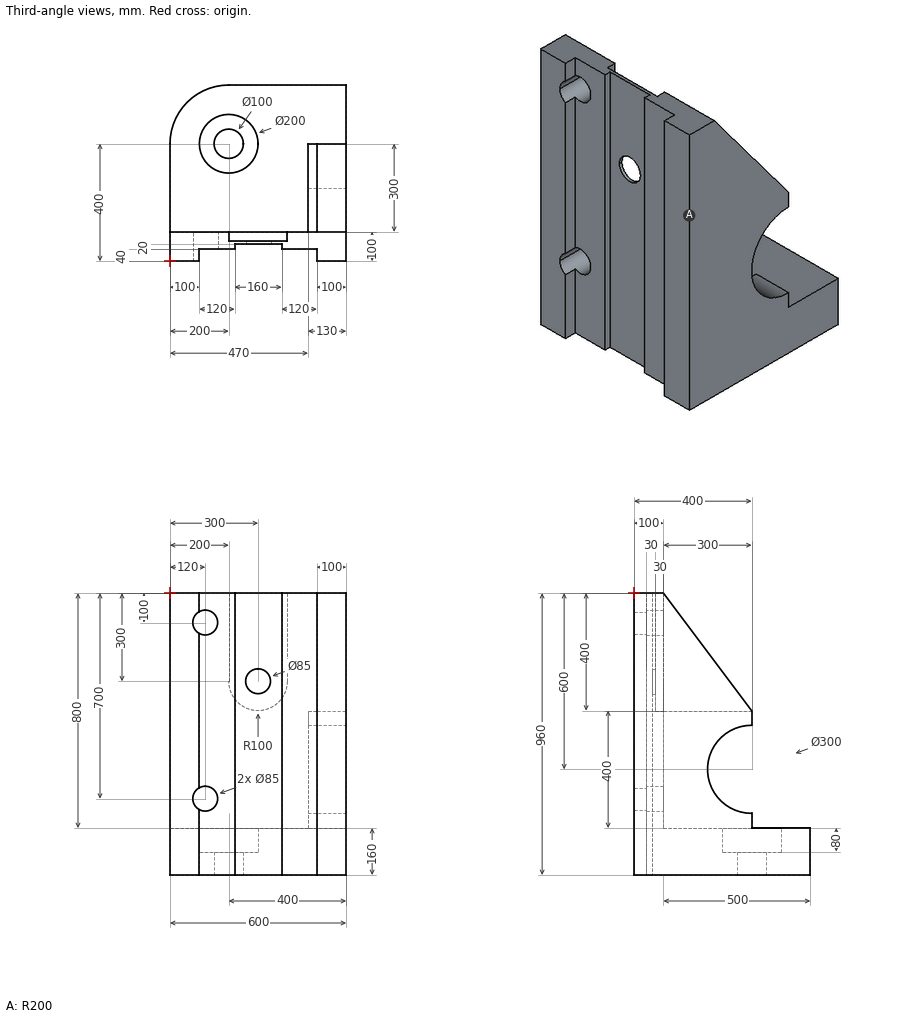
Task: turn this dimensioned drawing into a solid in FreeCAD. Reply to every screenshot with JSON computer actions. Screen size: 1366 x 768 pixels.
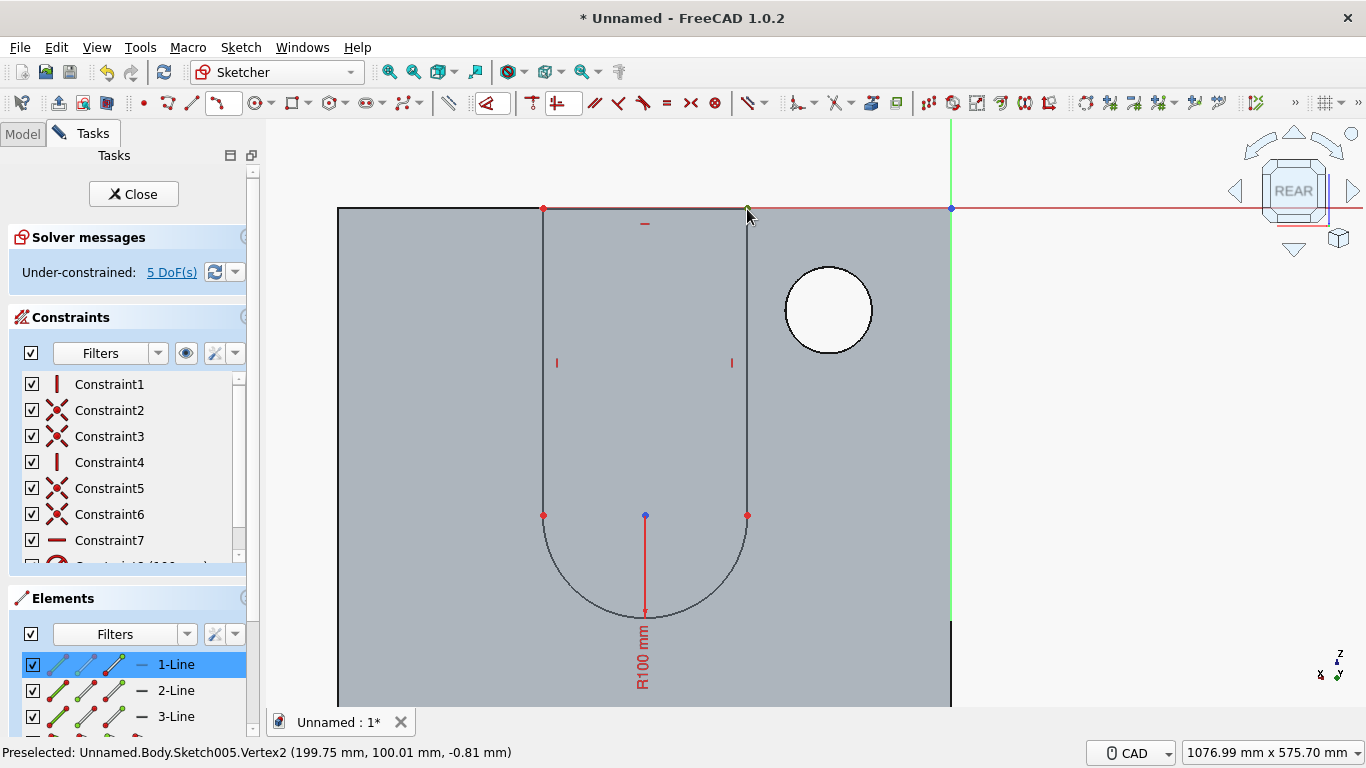
{"action": "left_click", "coordinate": [812, 208]}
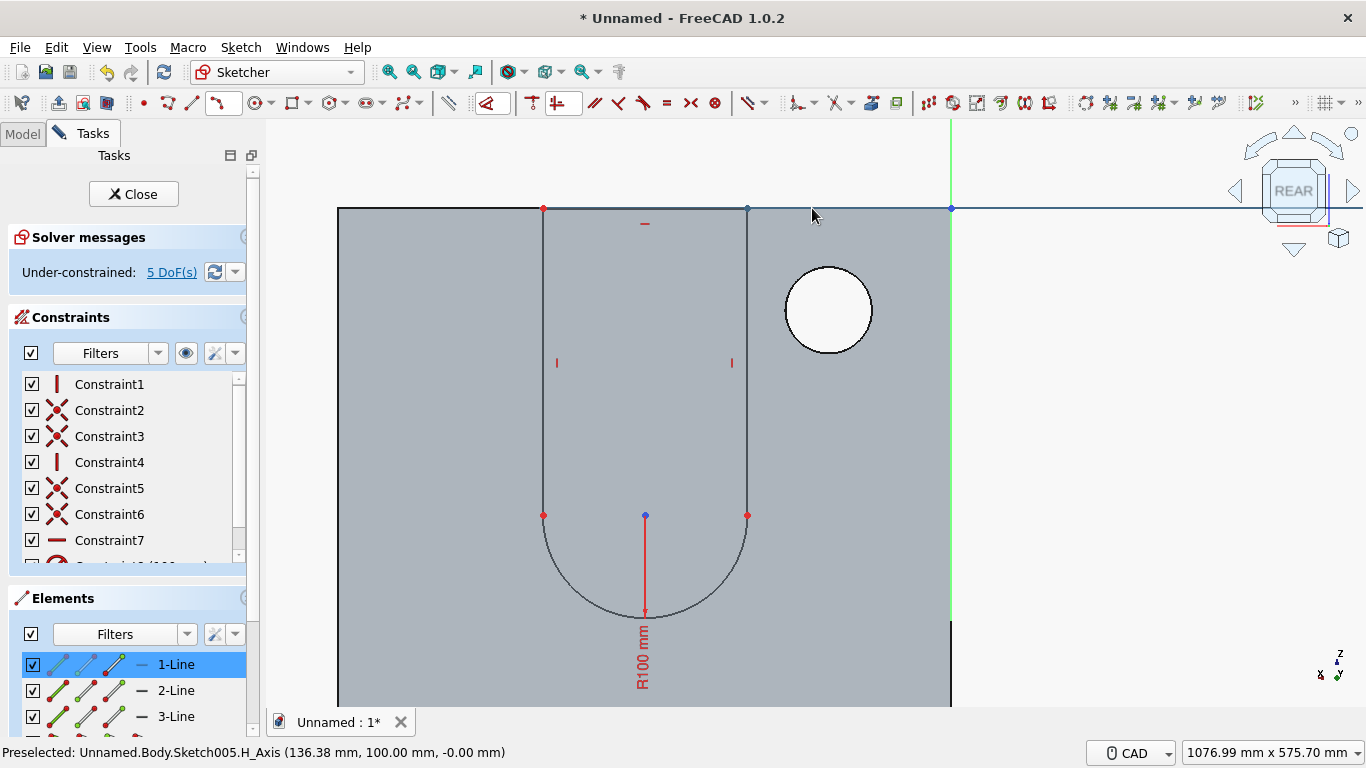
{"action": "left_click", "coordinate": [532, 104]}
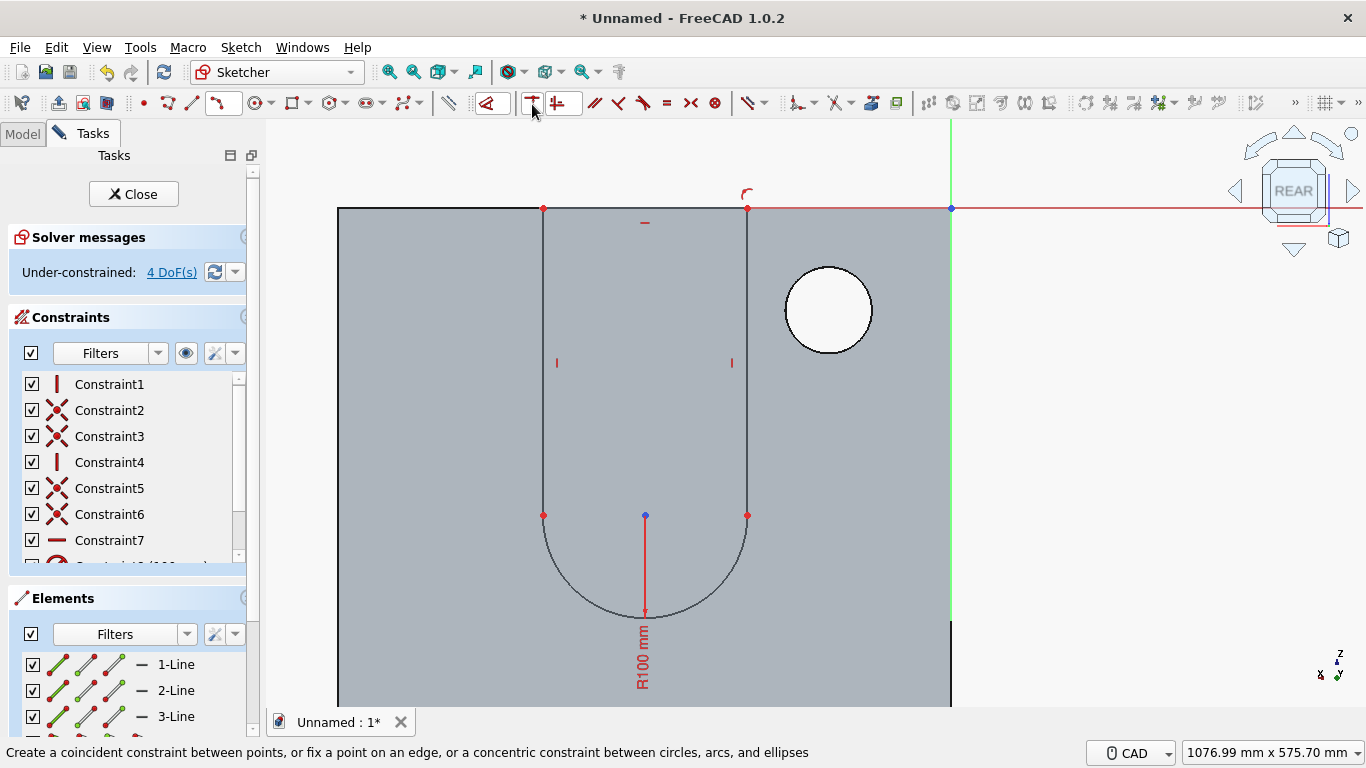
{"action": "left_click", "coordinate": [747, 424]}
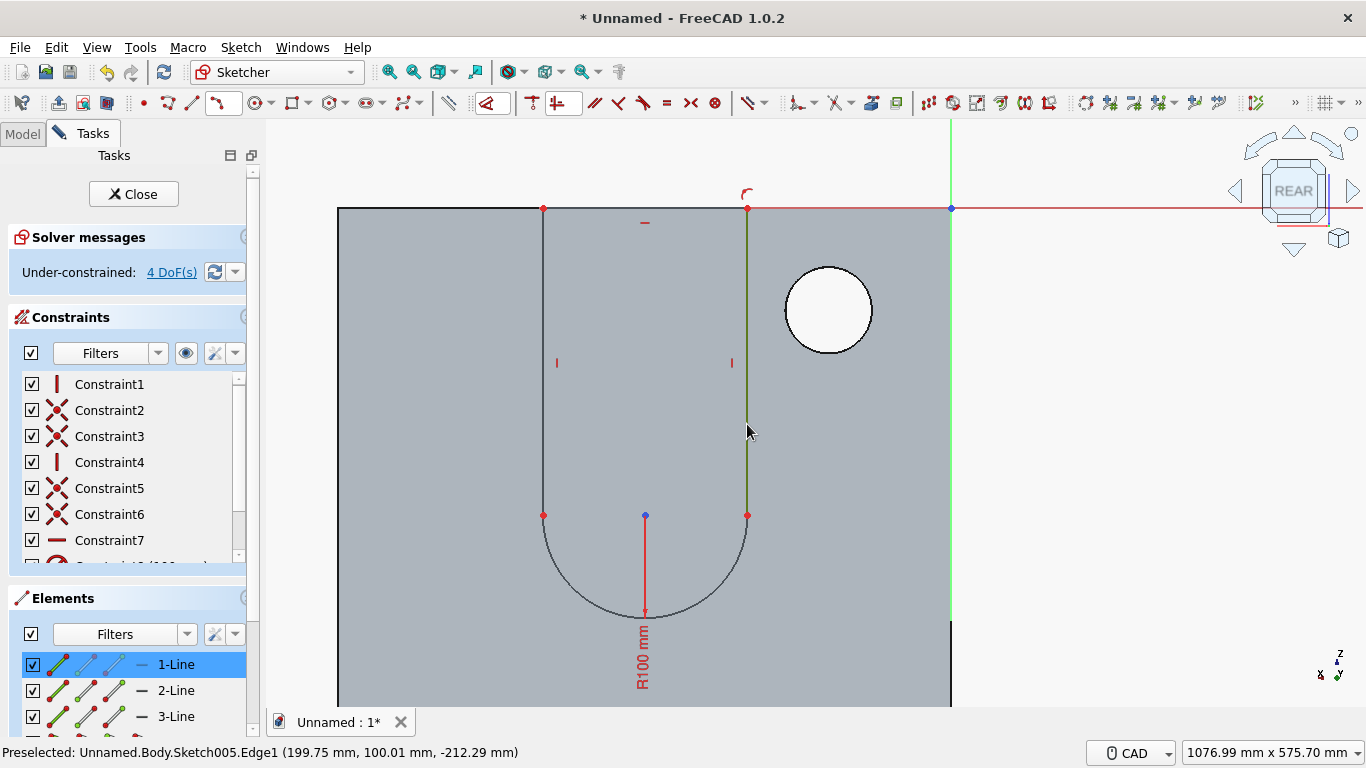
{"action": "key", "text": "i"}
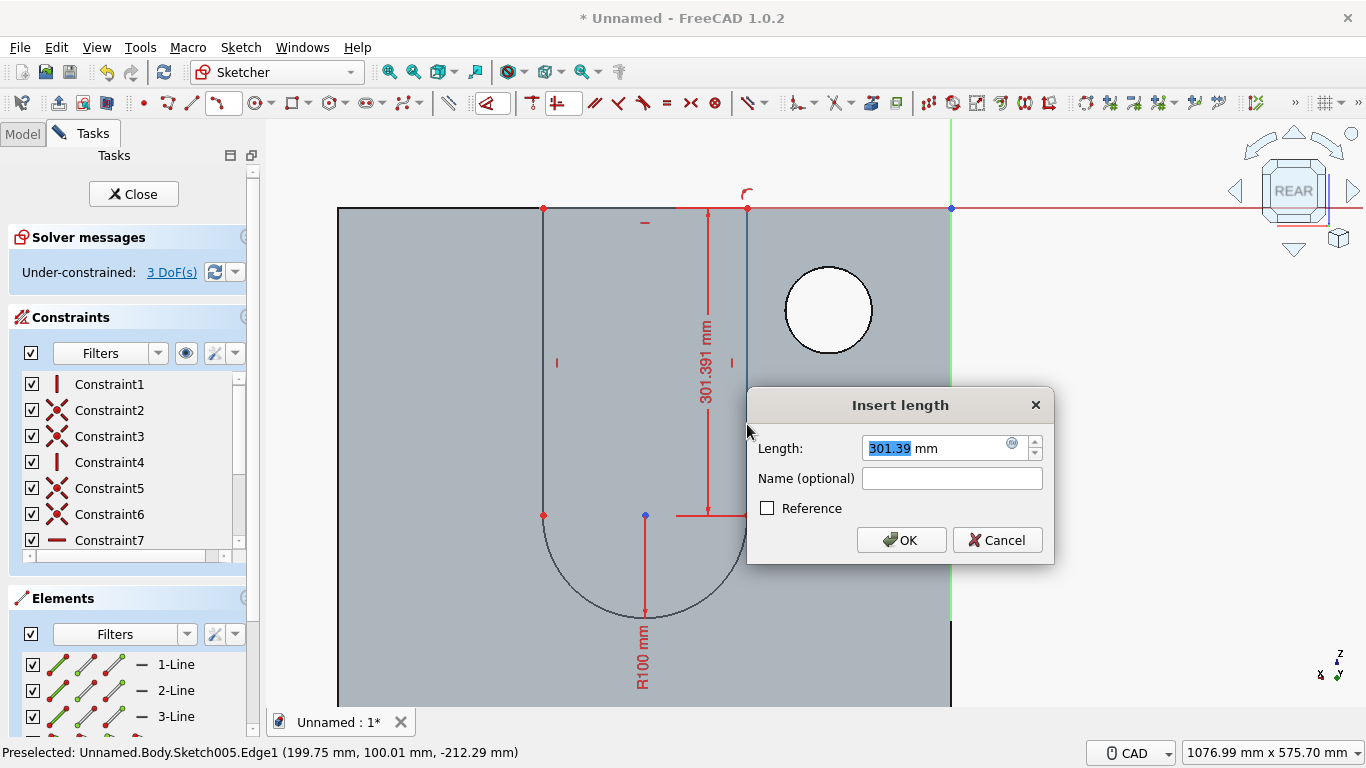
{"action": "type", "text": "300"}
{"action": "key", "text": "Return"}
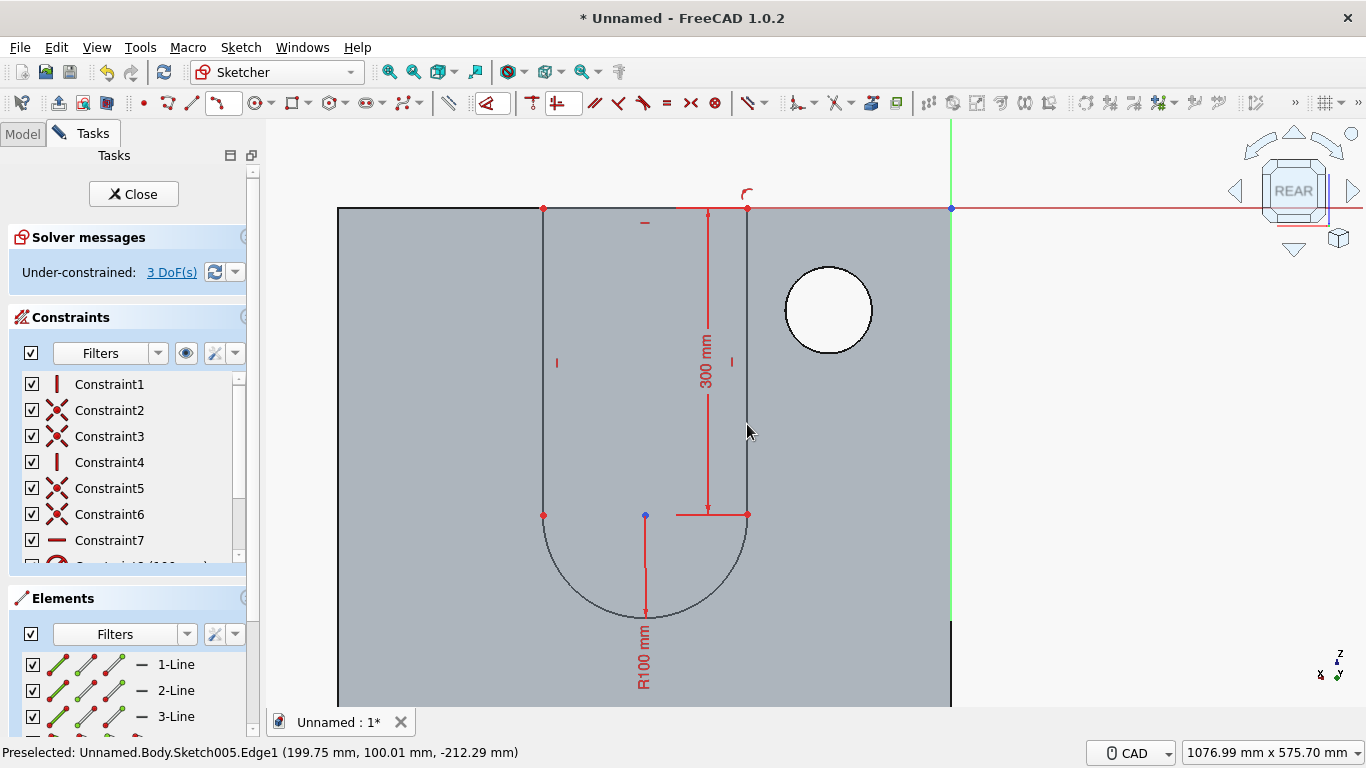
{"action": "left_click", "coordinate": [543, 301]}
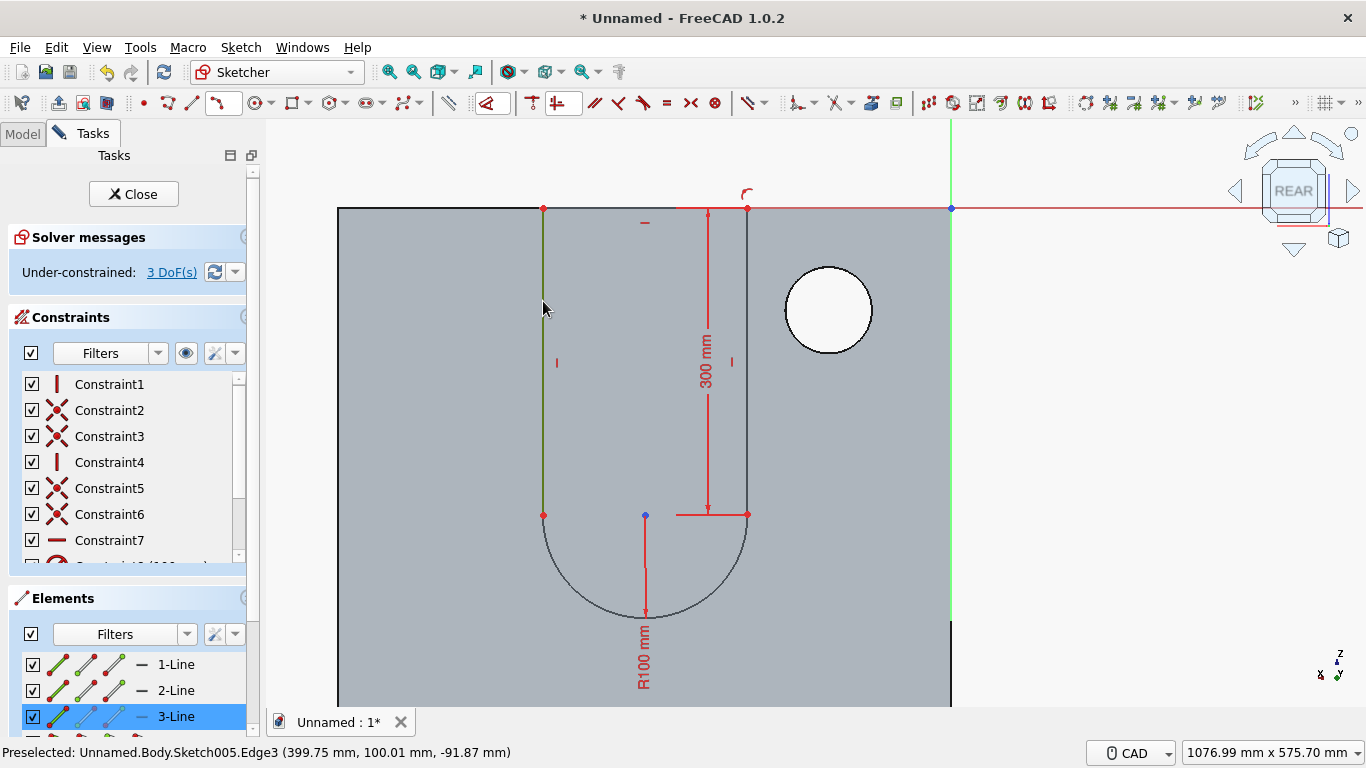
{"action": "left_click", "coordinate": [504, 104]}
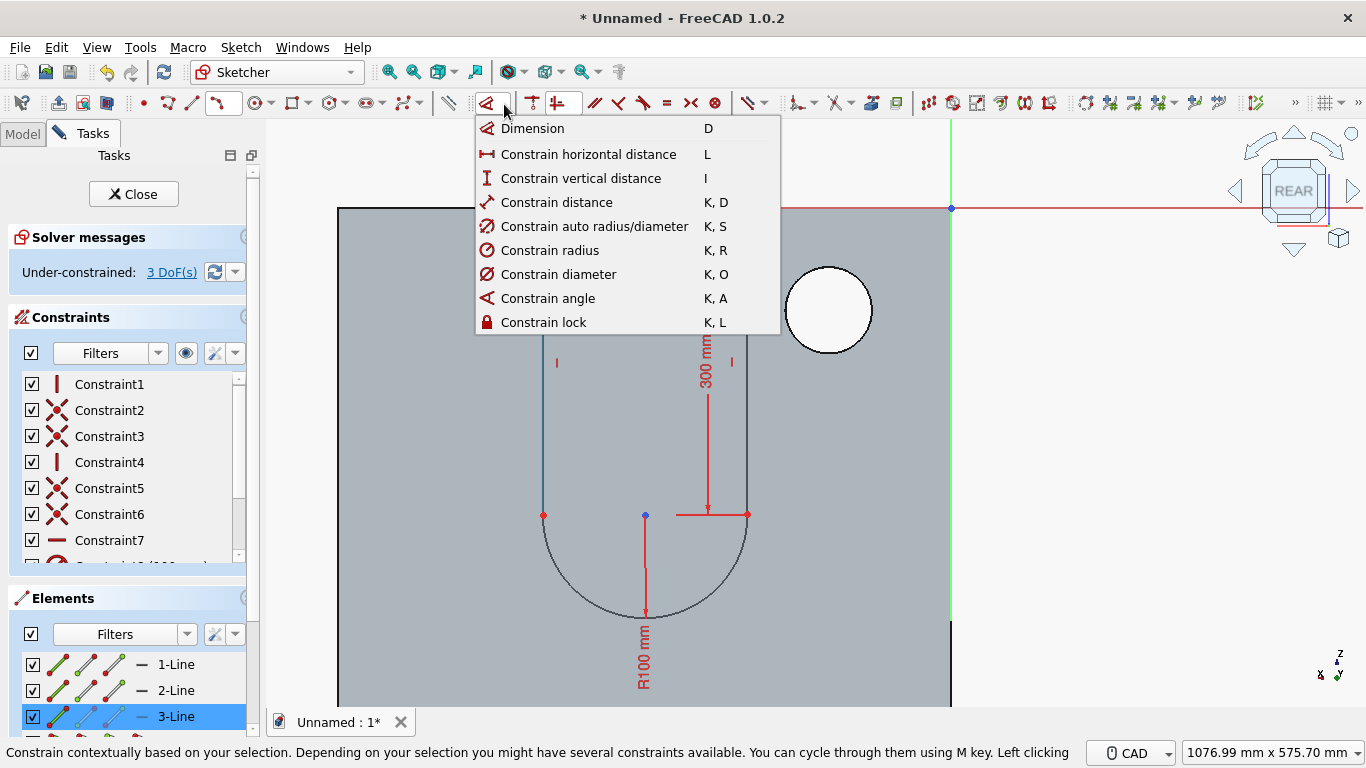
{"action": "left_click", "coordinate": [628, 178]}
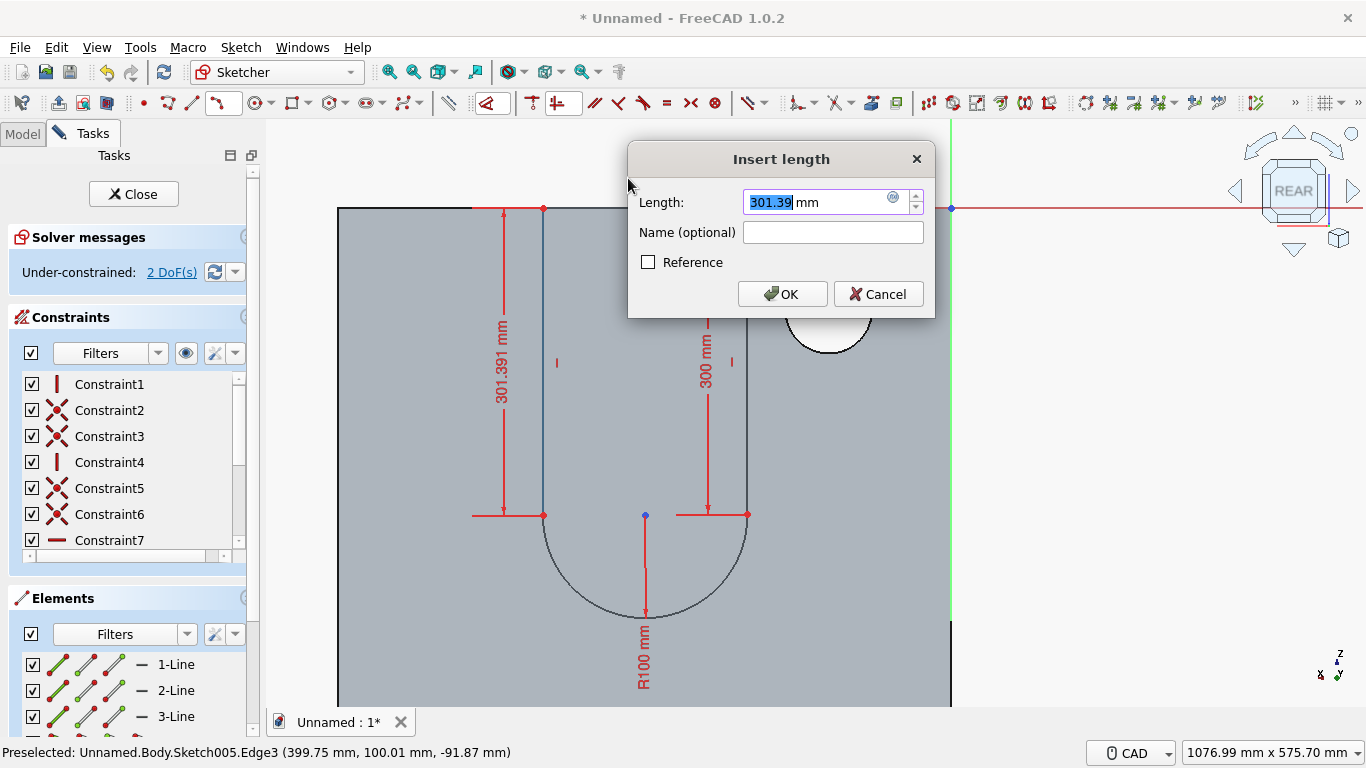
{"action": "type", "text": "300"}
{"action": "key", "text": "Return"}